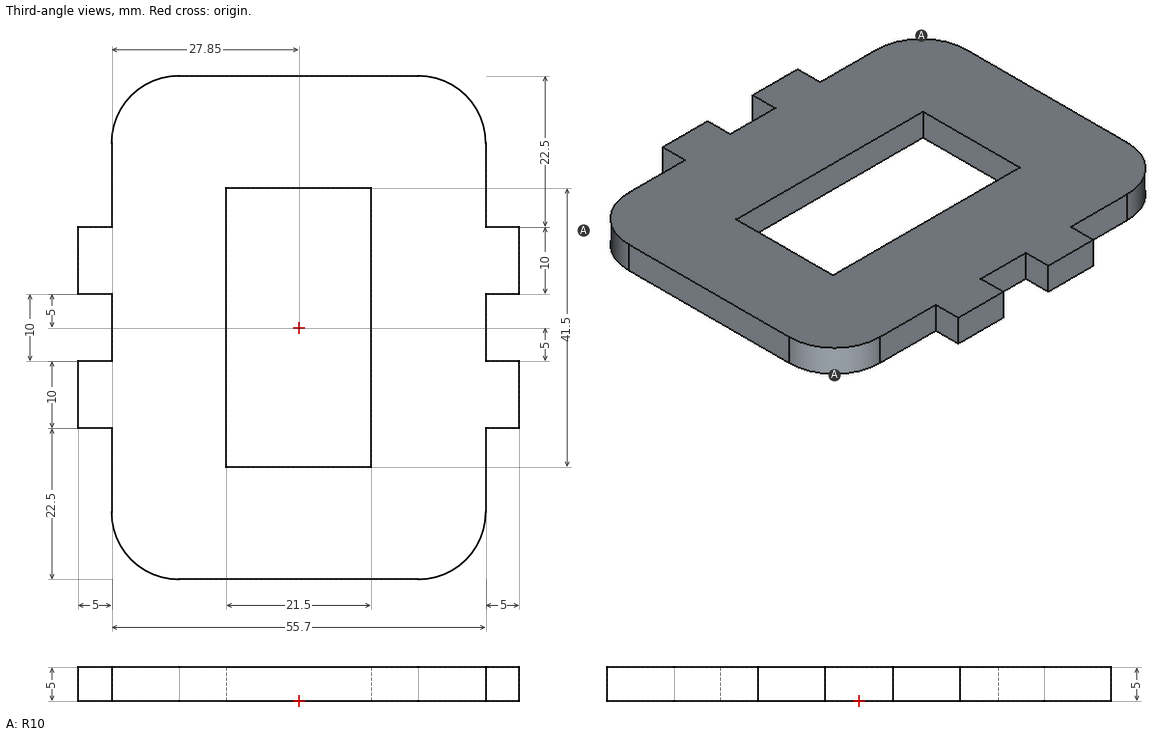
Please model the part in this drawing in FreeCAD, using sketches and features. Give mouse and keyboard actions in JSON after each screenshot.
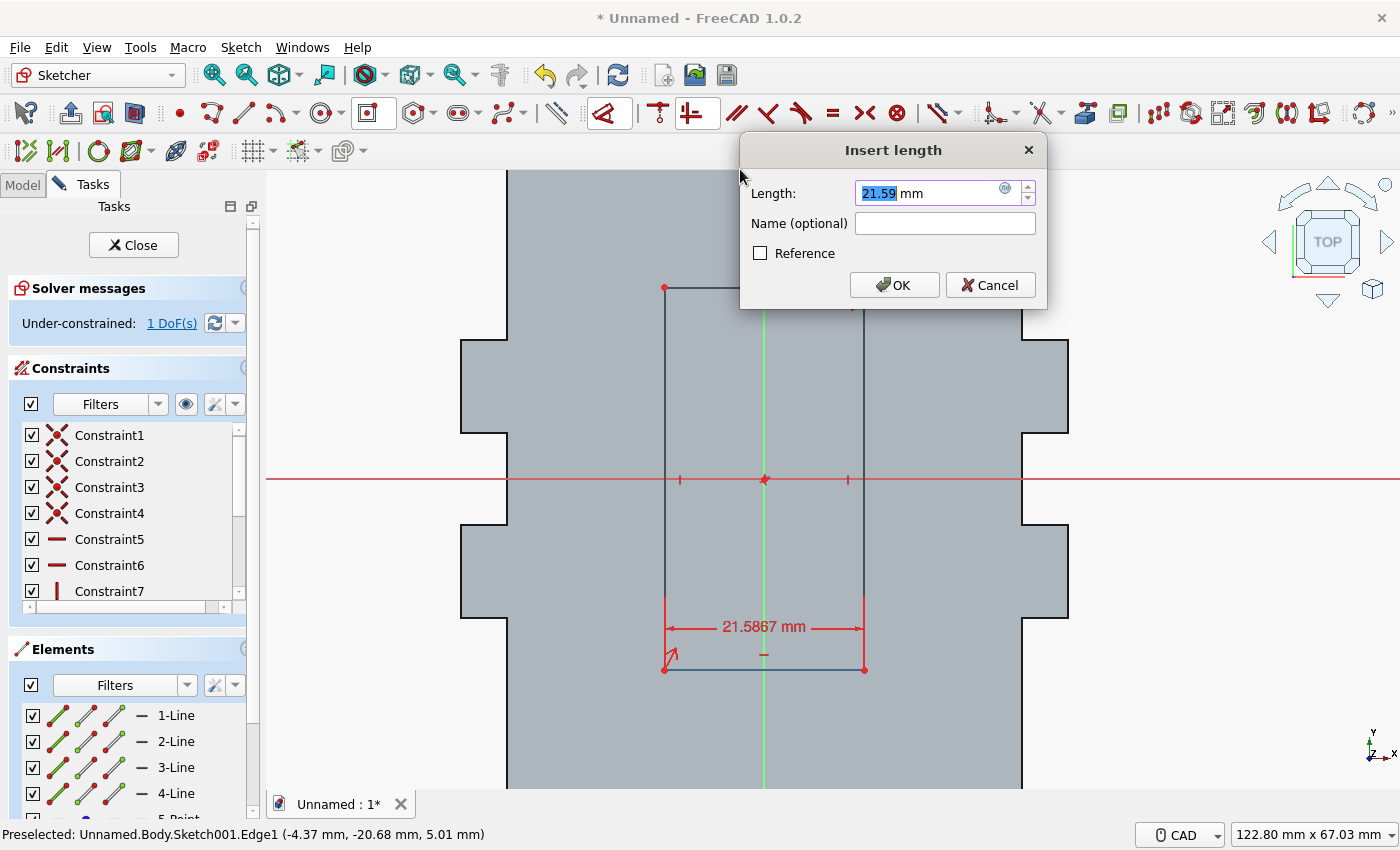
{"action": "type", "text": "21.5"}
{"action": "key", "text": "Return"}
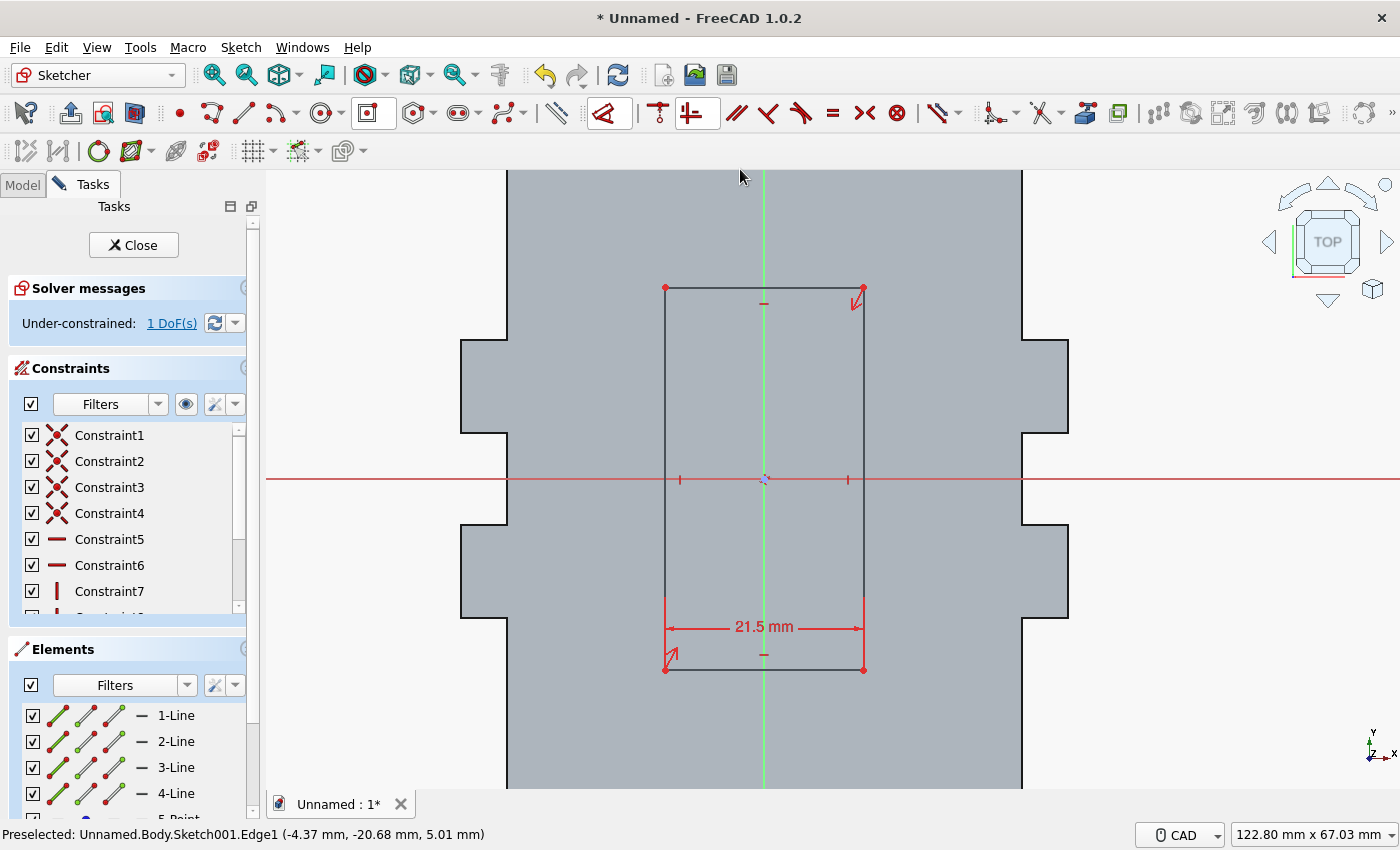
{"action": "left_click", "coordinate": [864, 555]}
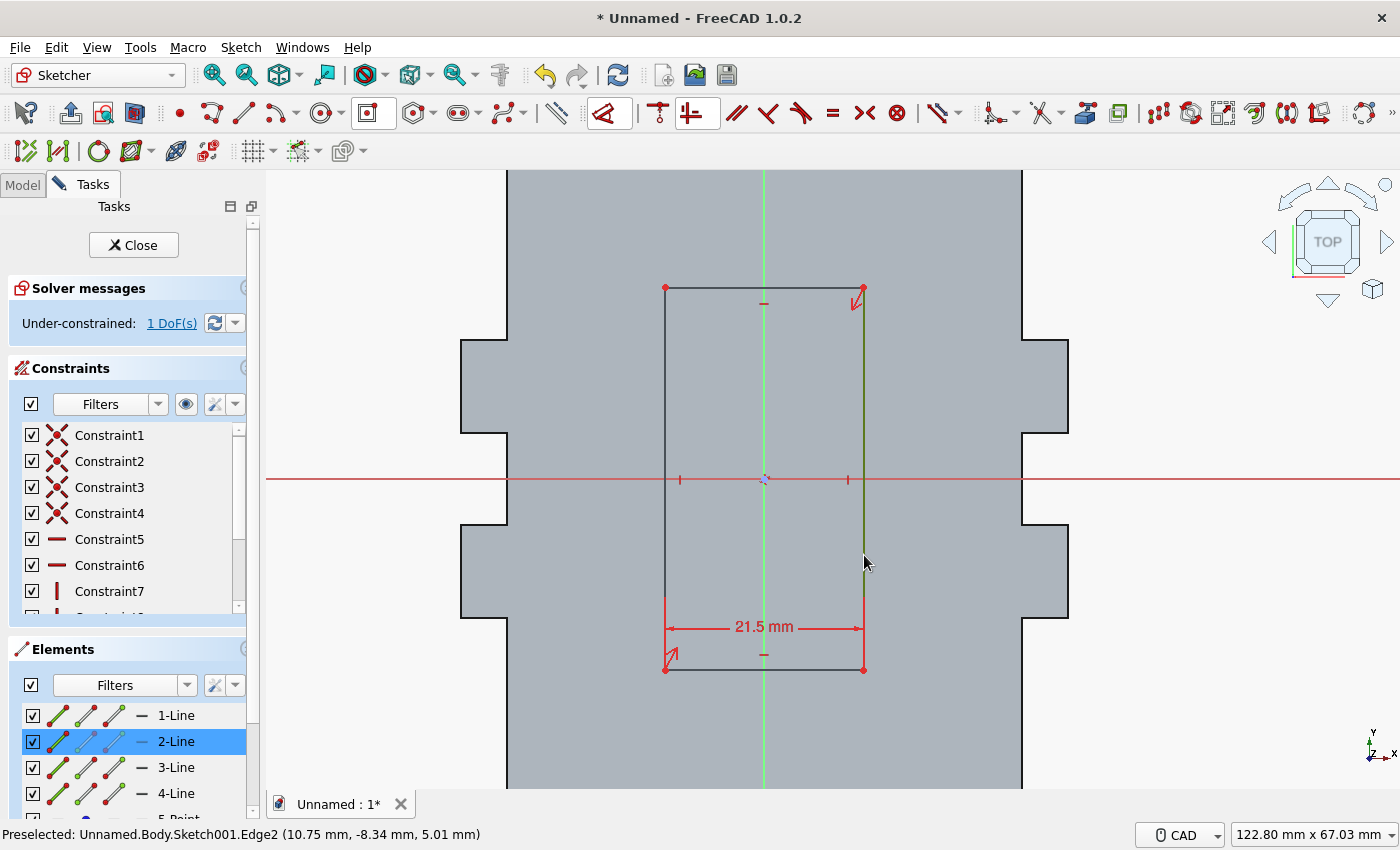
{"action": "key", "text": "i"}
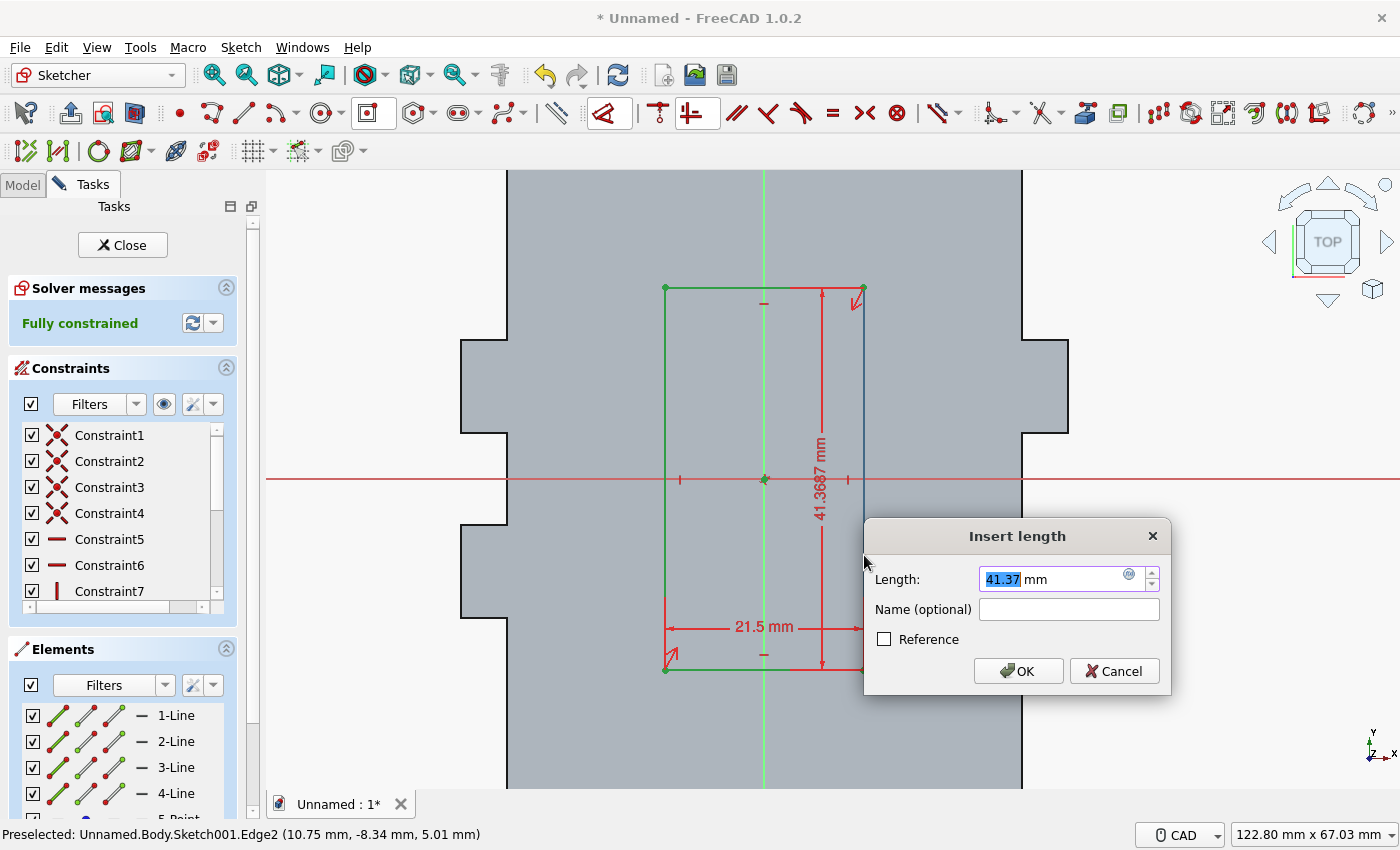
{"action": "type", "text": "41.5"}
{"action": "key", "text": "Return"}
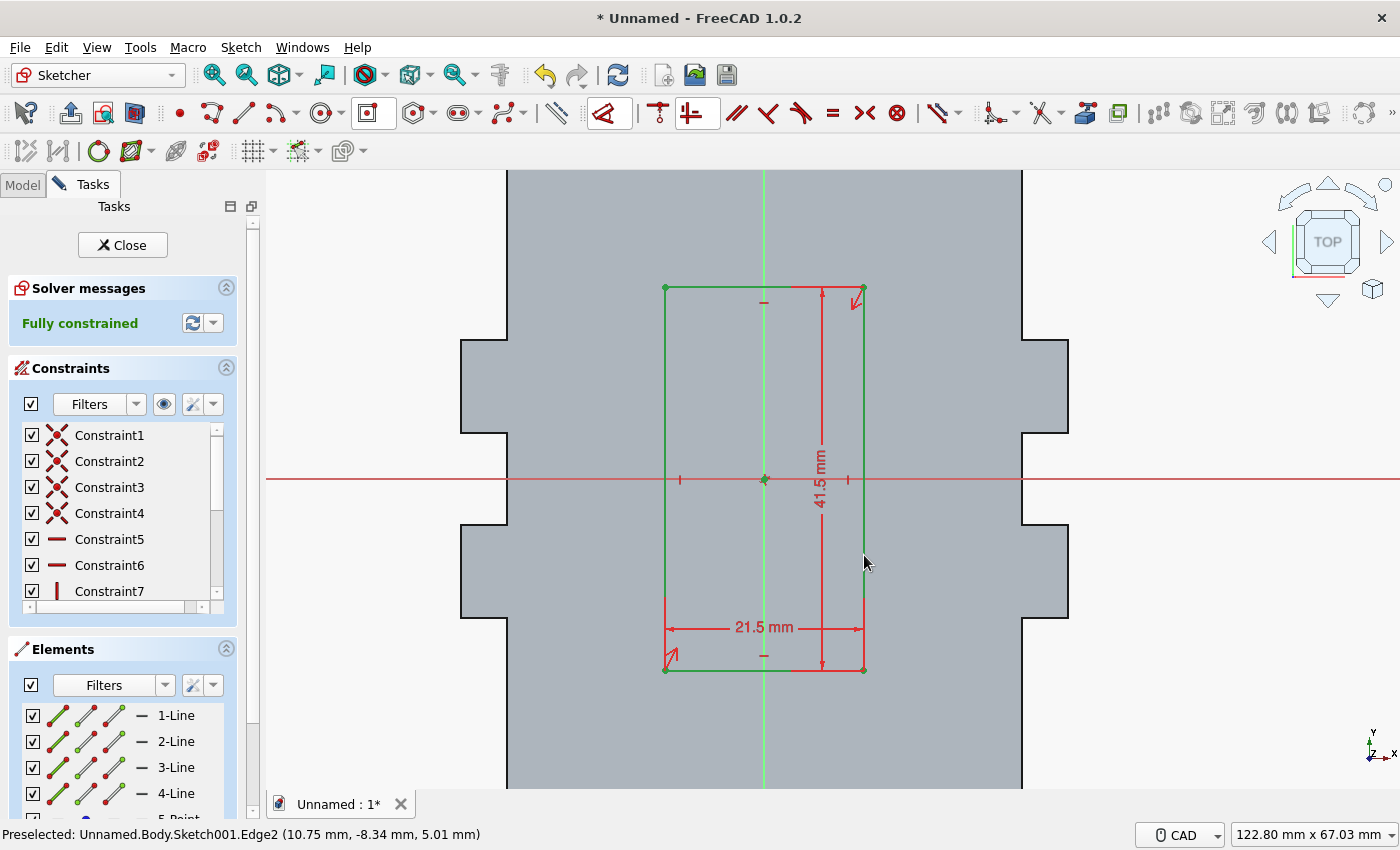
{"action": "left_click", "coordinate": [123, 245]}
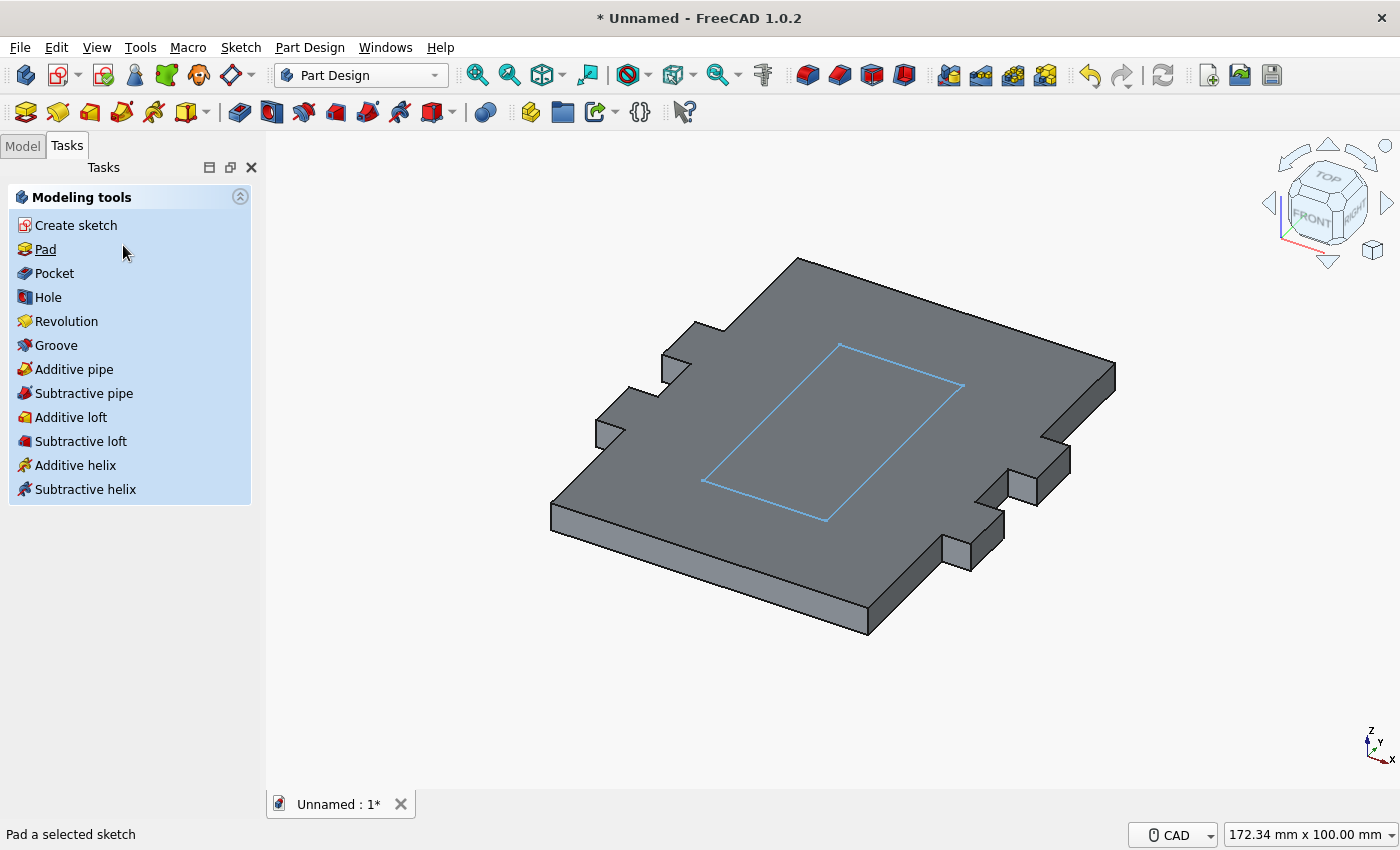
{"action": "left_click", "coordinate": [240, 112]}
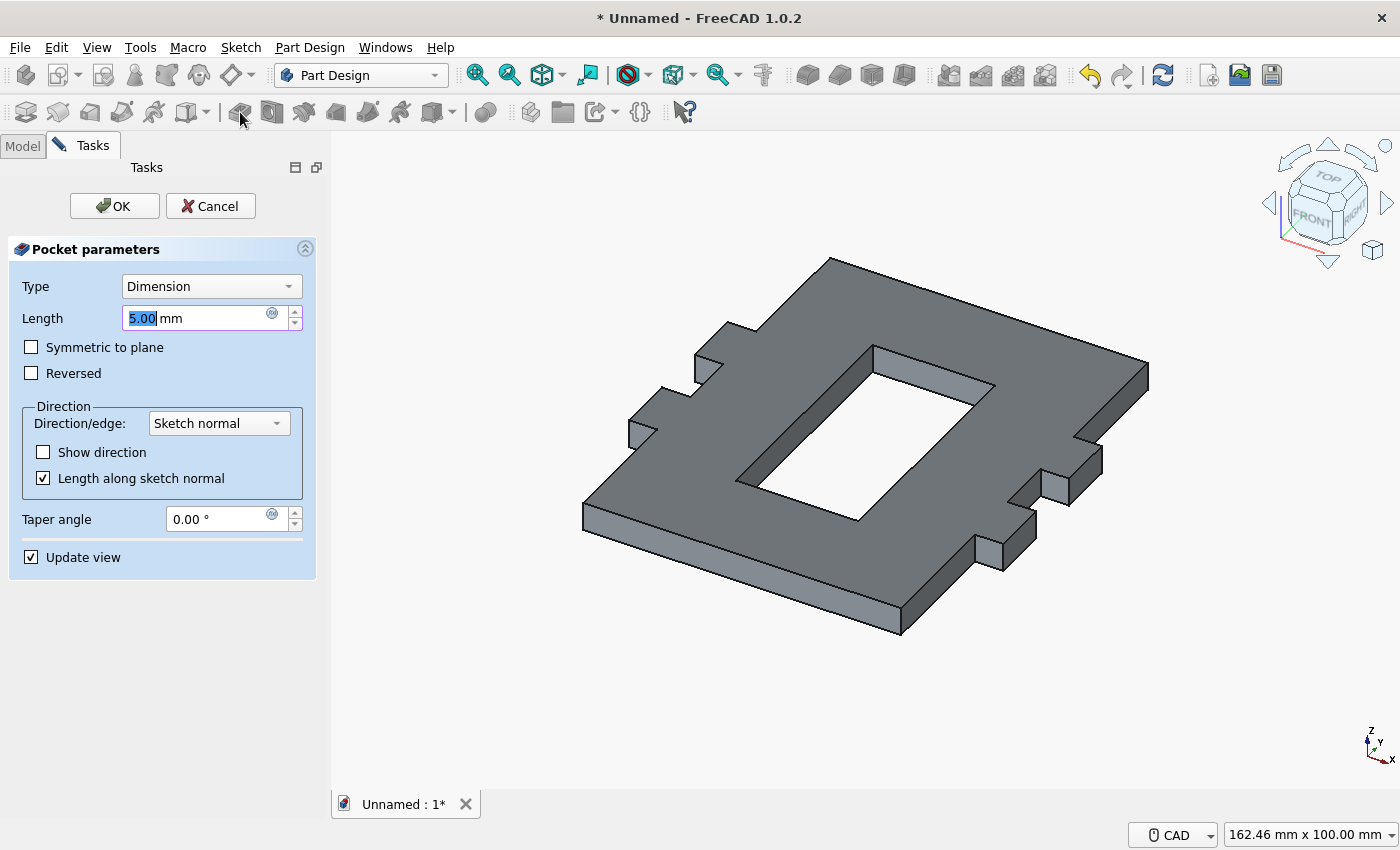
{"action": "type", "text": "5"}
{"action": "key", "text": "Tab"}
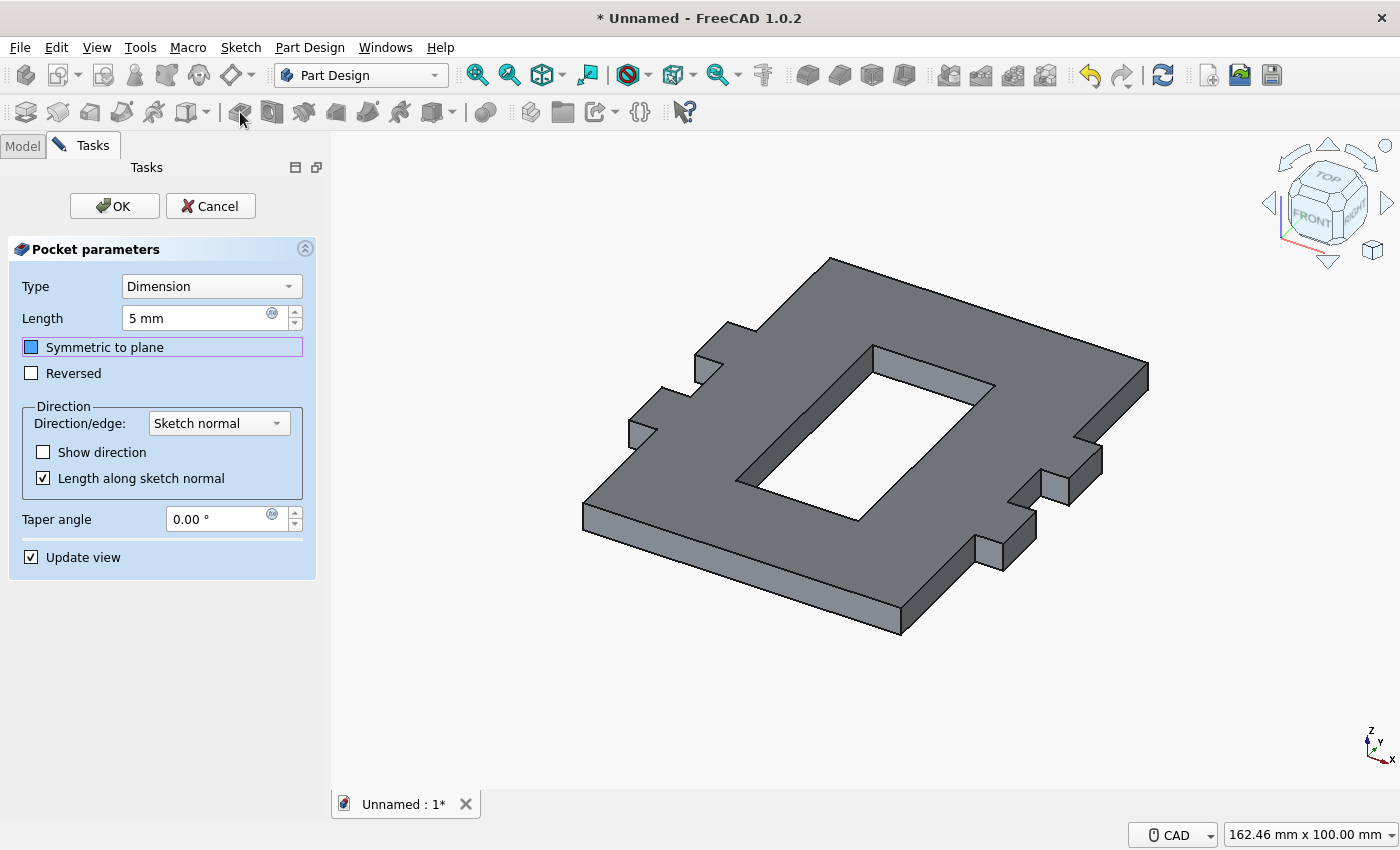
{"action": "left_click", "coordinate": [115, 206]}